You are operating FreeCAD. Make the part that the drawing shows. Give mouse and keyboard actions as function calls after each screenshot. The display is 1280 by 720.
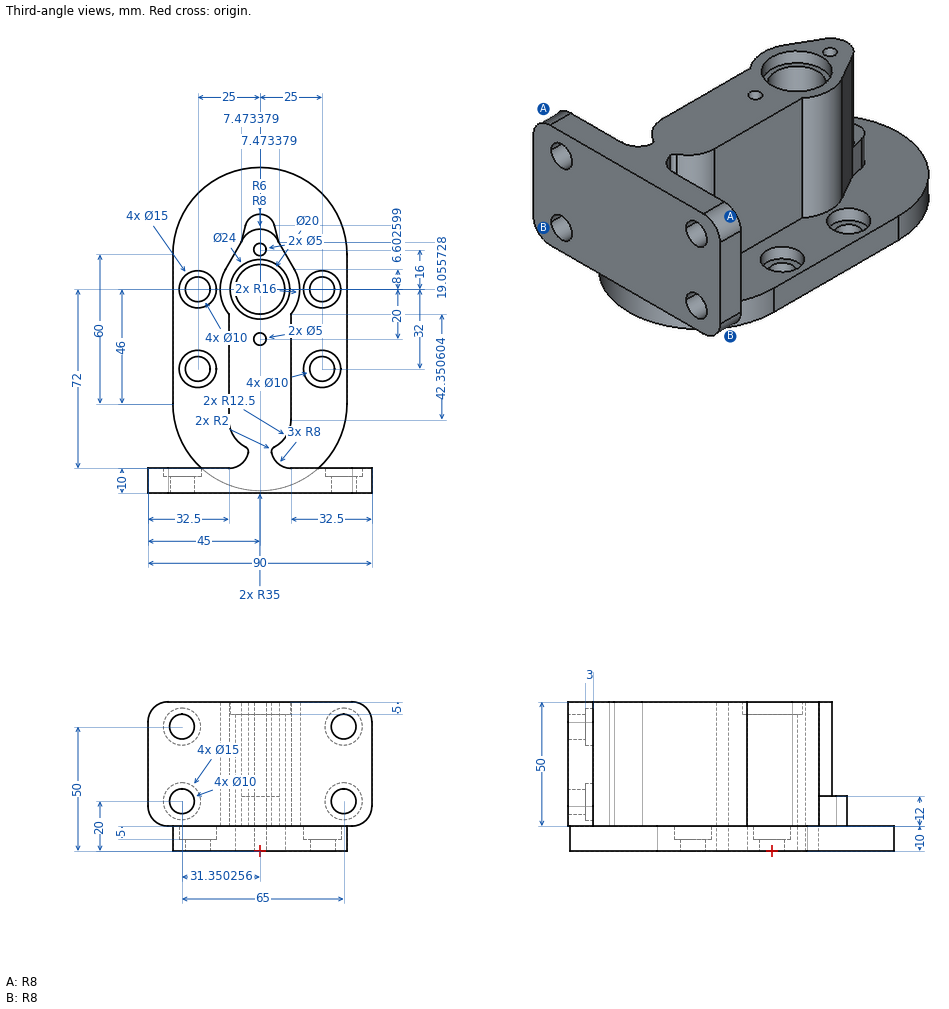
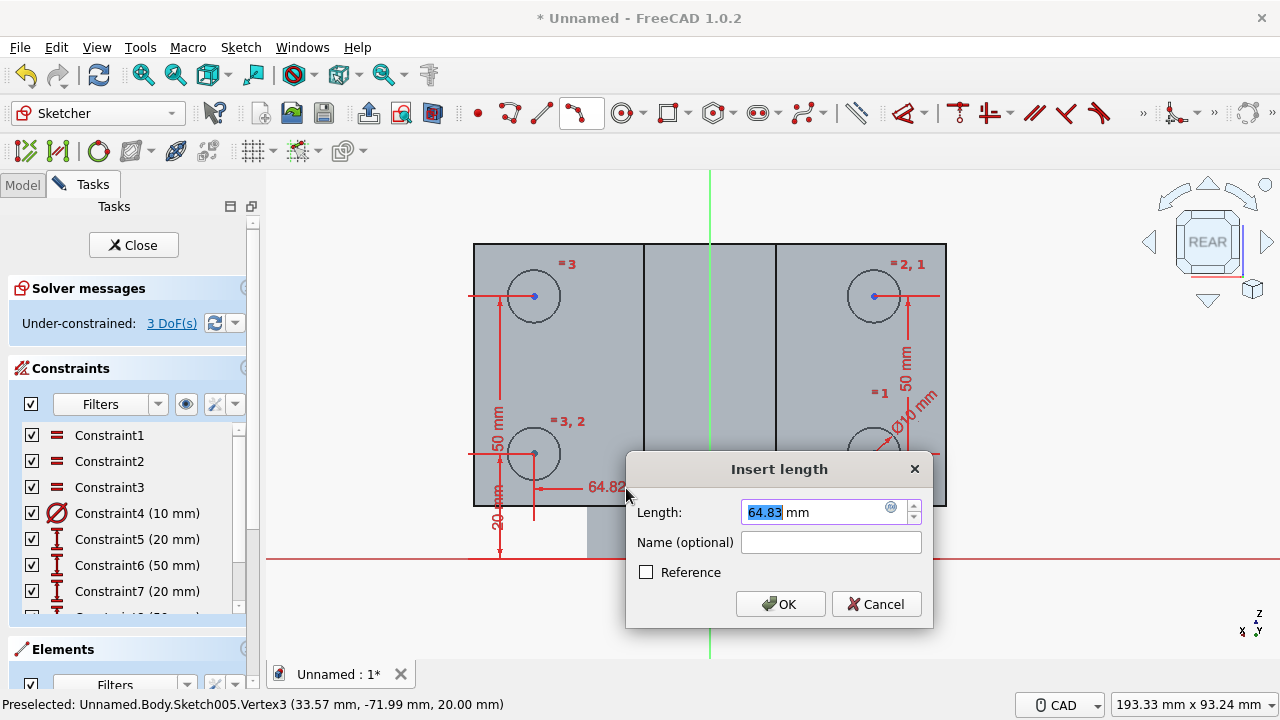
text(65)
key(Return)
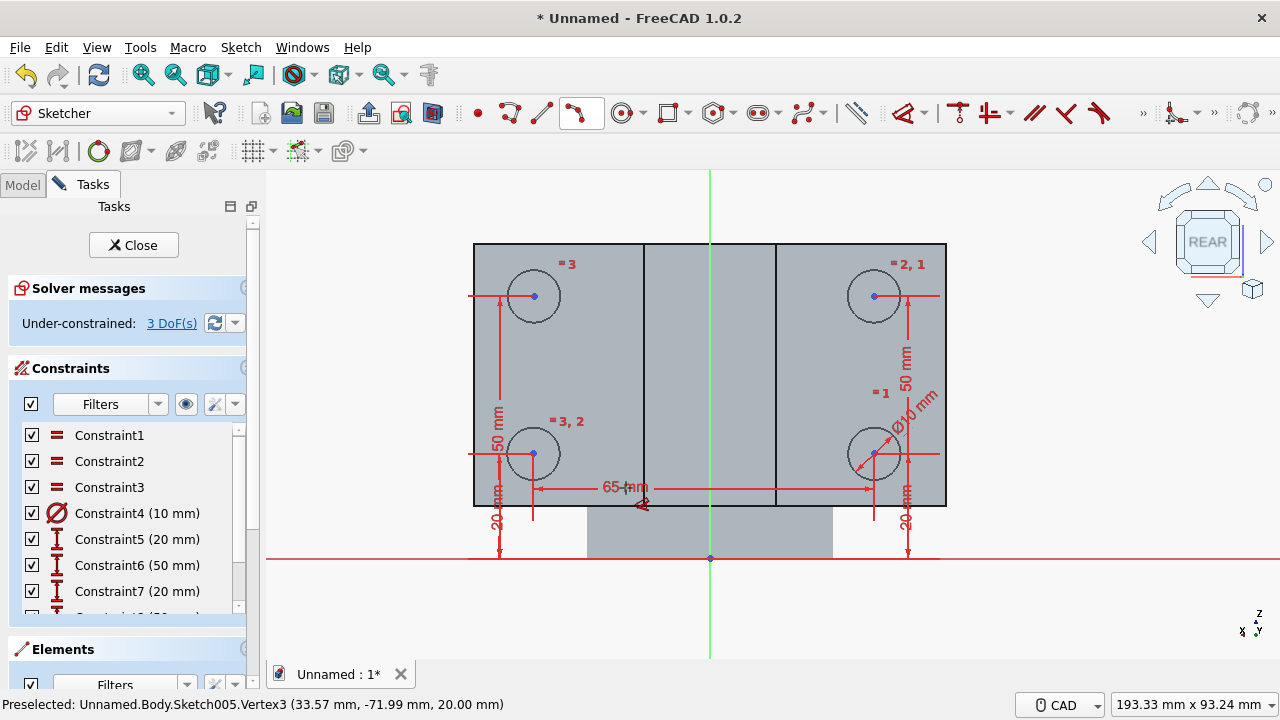
click(874, 296)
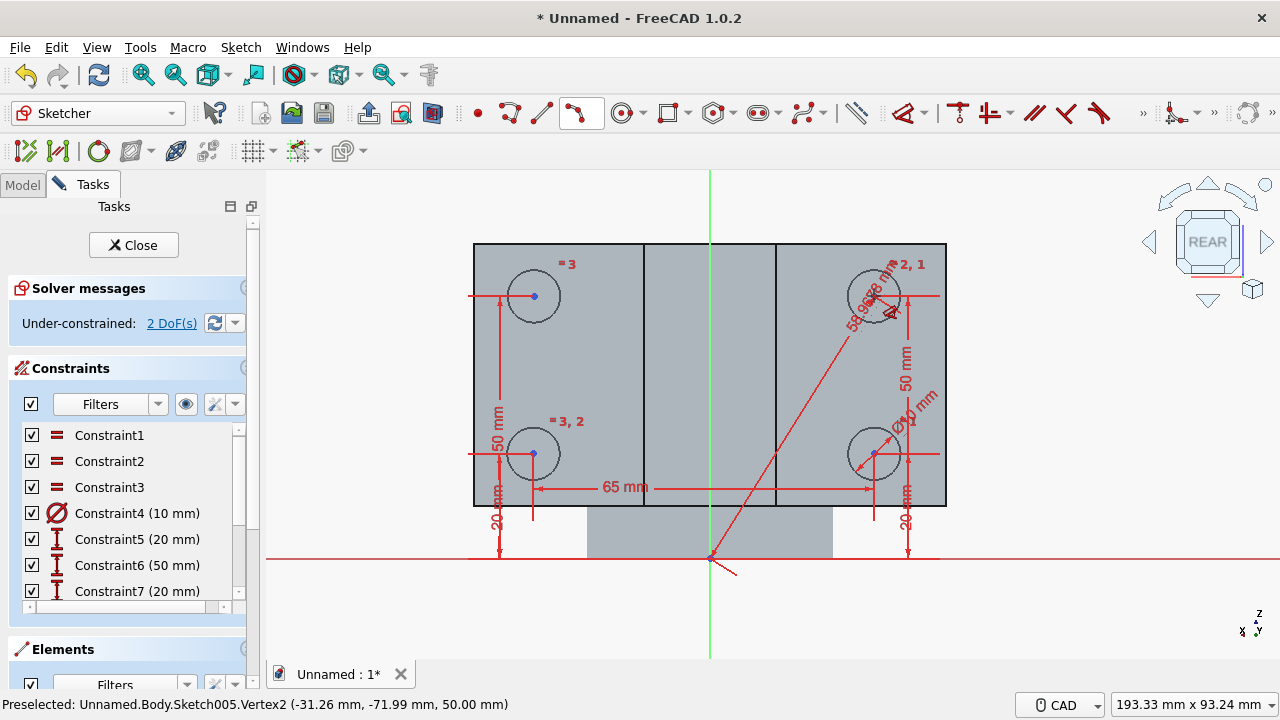
click(533, 454)
click(625, 262)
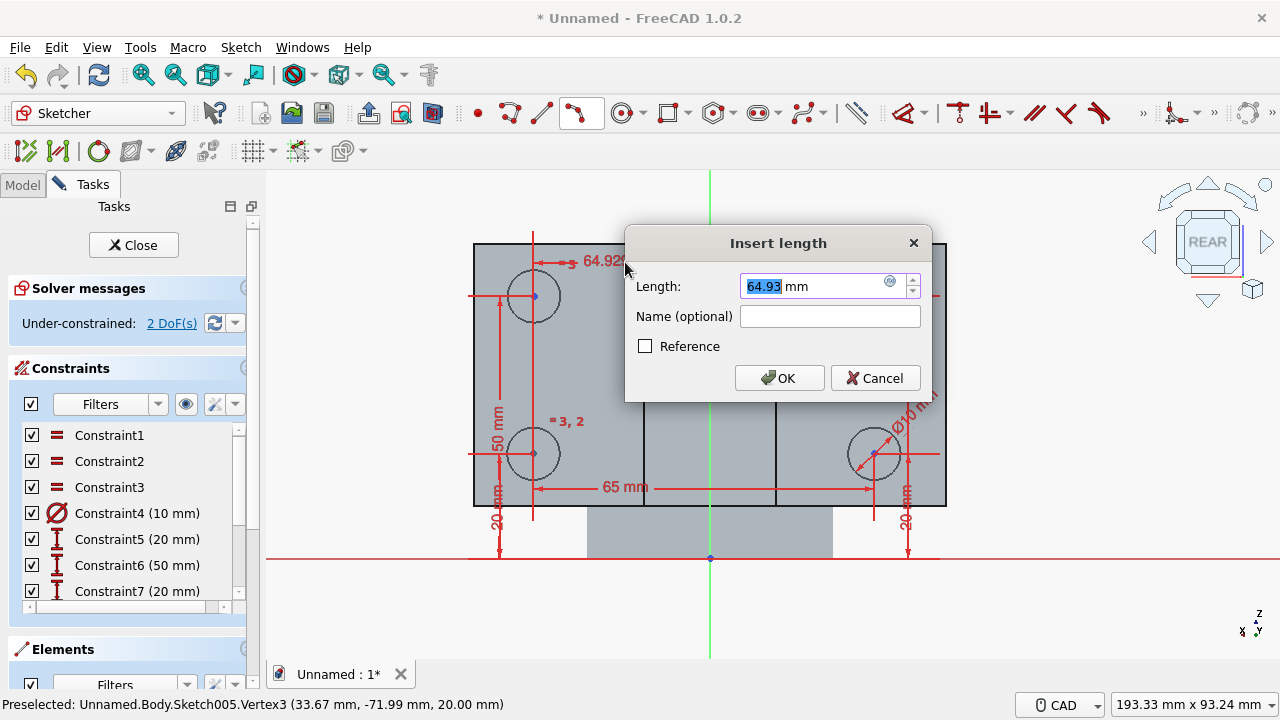
text(65)
key(Return)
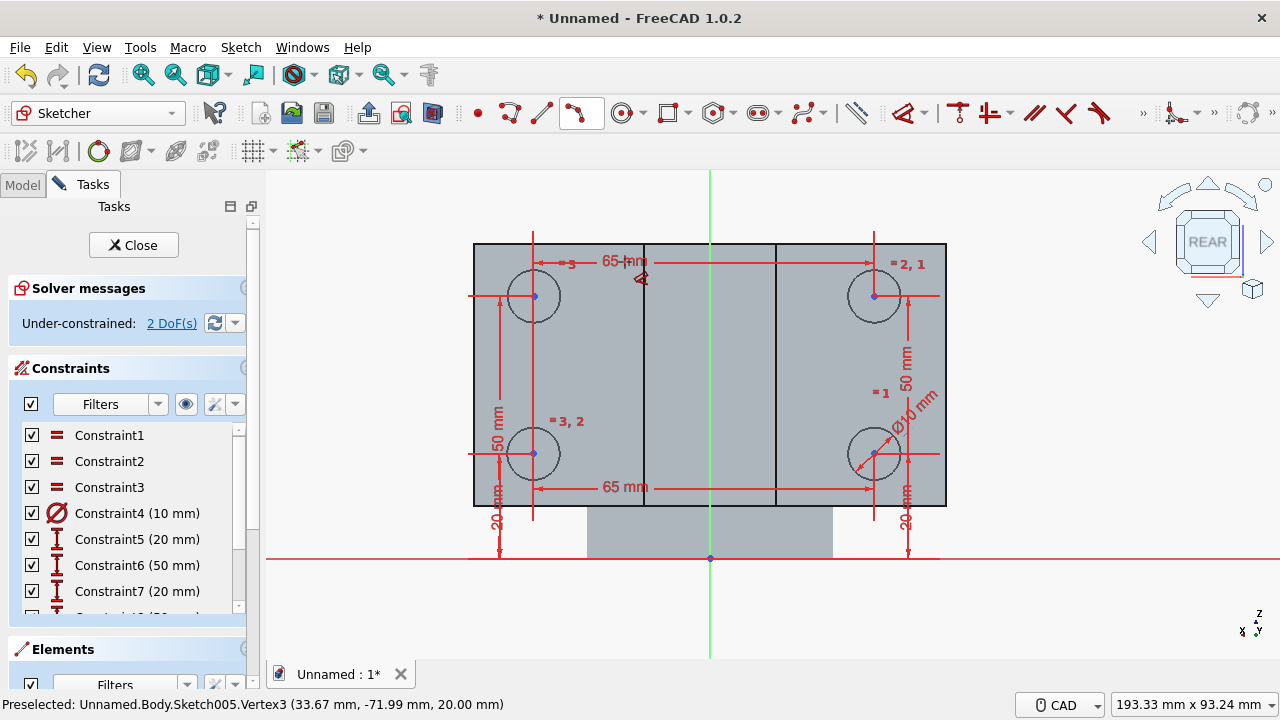
click(874, 296)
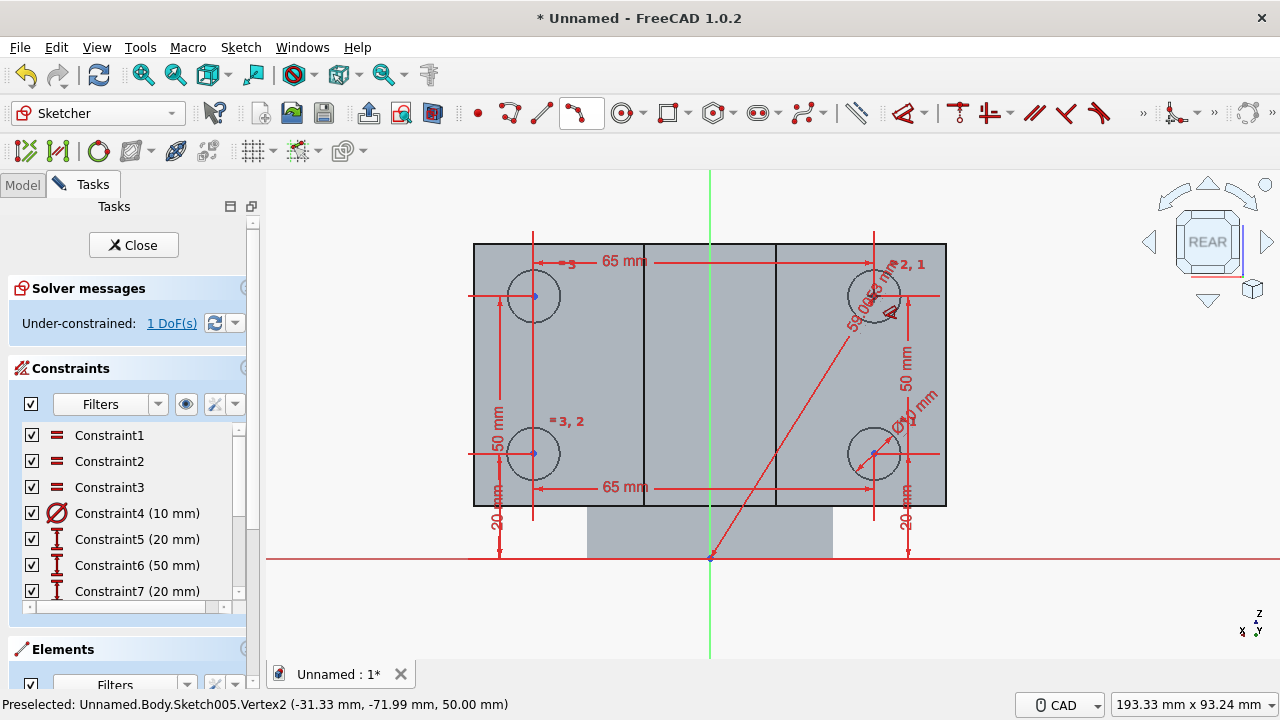
click(534, 296)
click(782, 262)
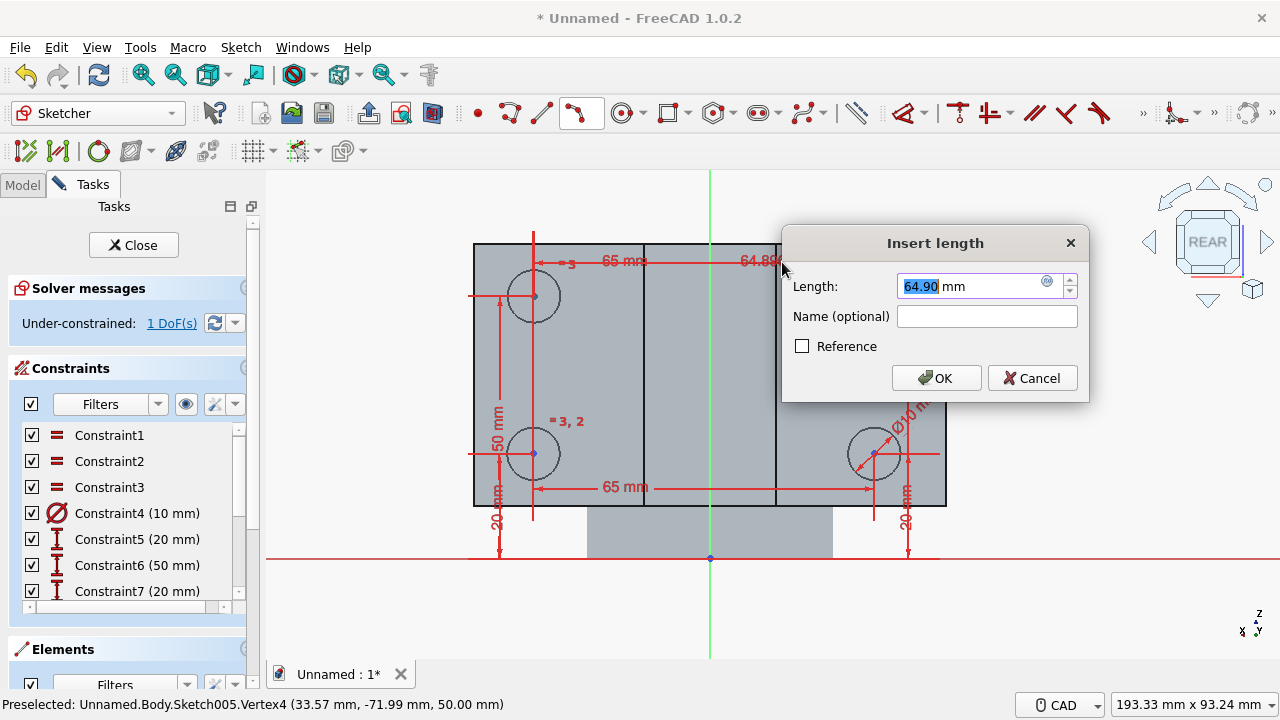
text(65)
key(Return)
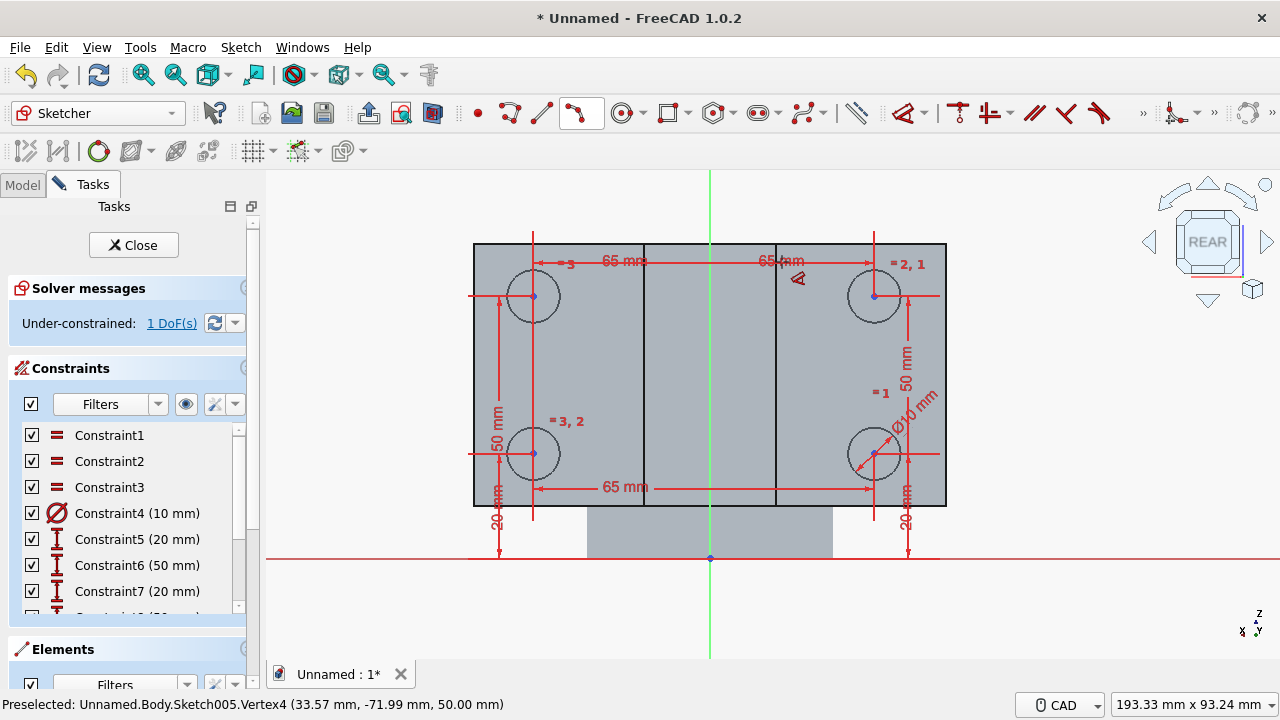
click(874, 454)
click(792, 593)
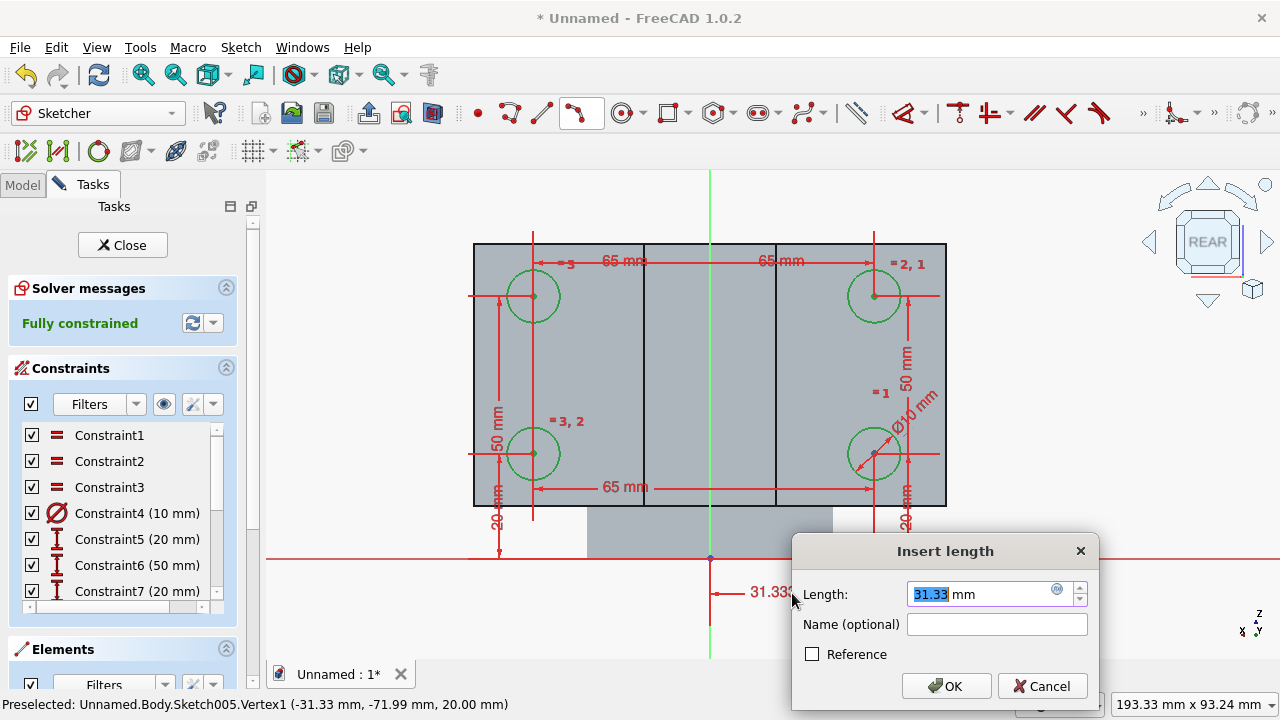
text(31.350256)
key(Return)
key(Escape)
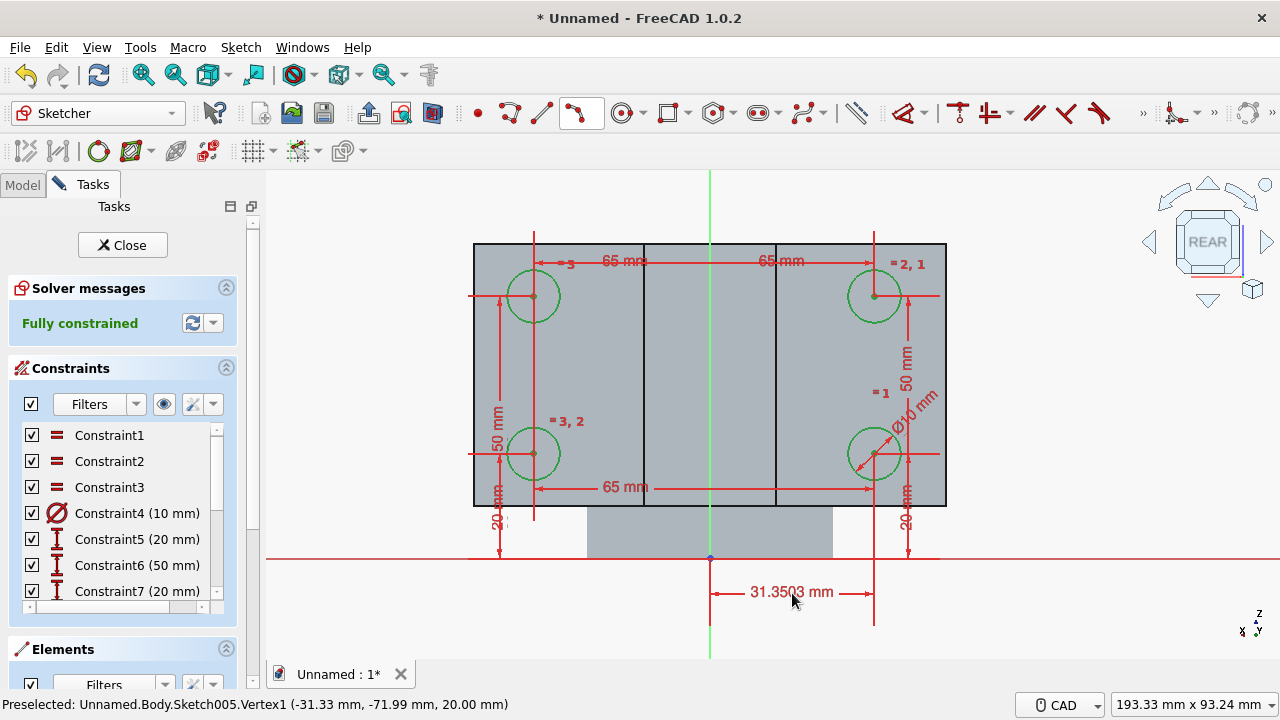
click(123, 245)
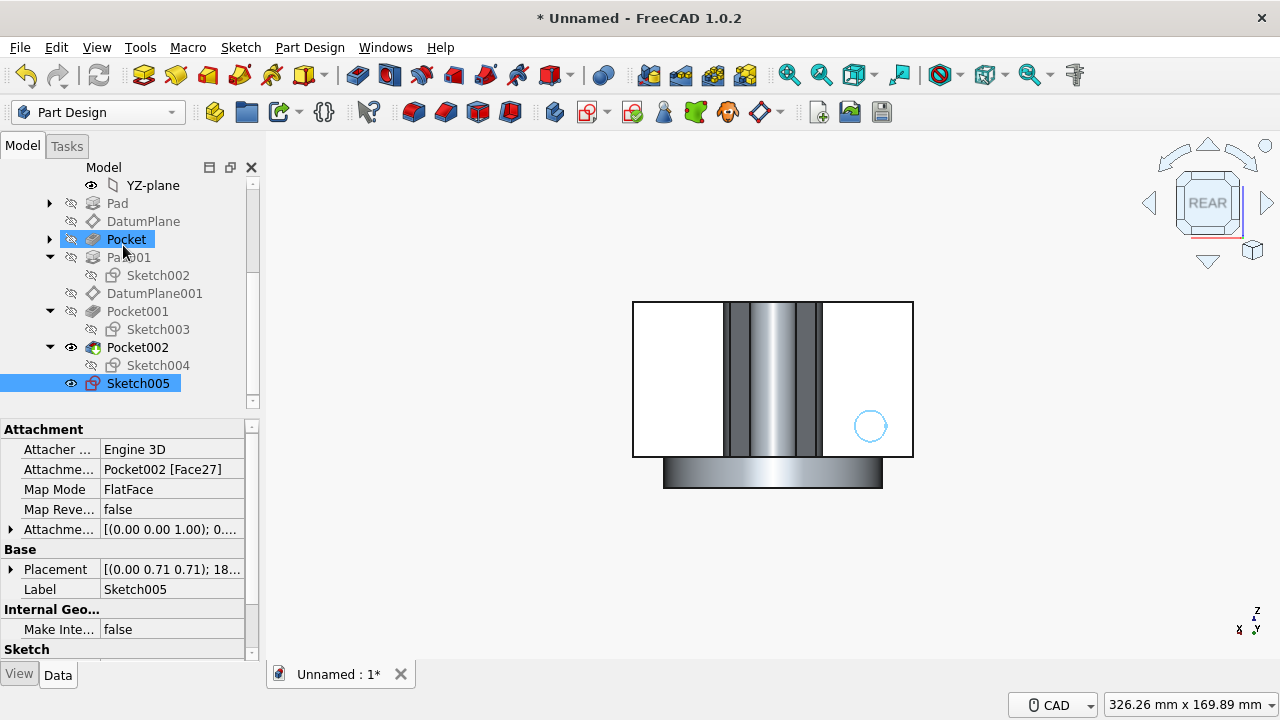
click(358, 76)